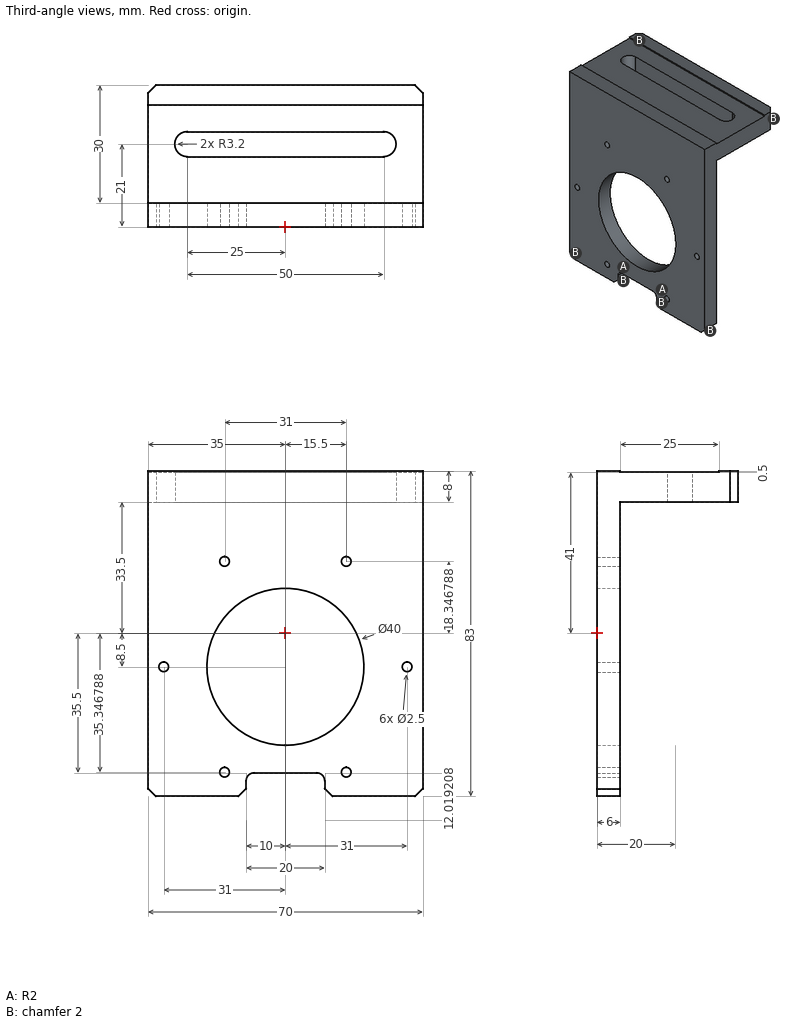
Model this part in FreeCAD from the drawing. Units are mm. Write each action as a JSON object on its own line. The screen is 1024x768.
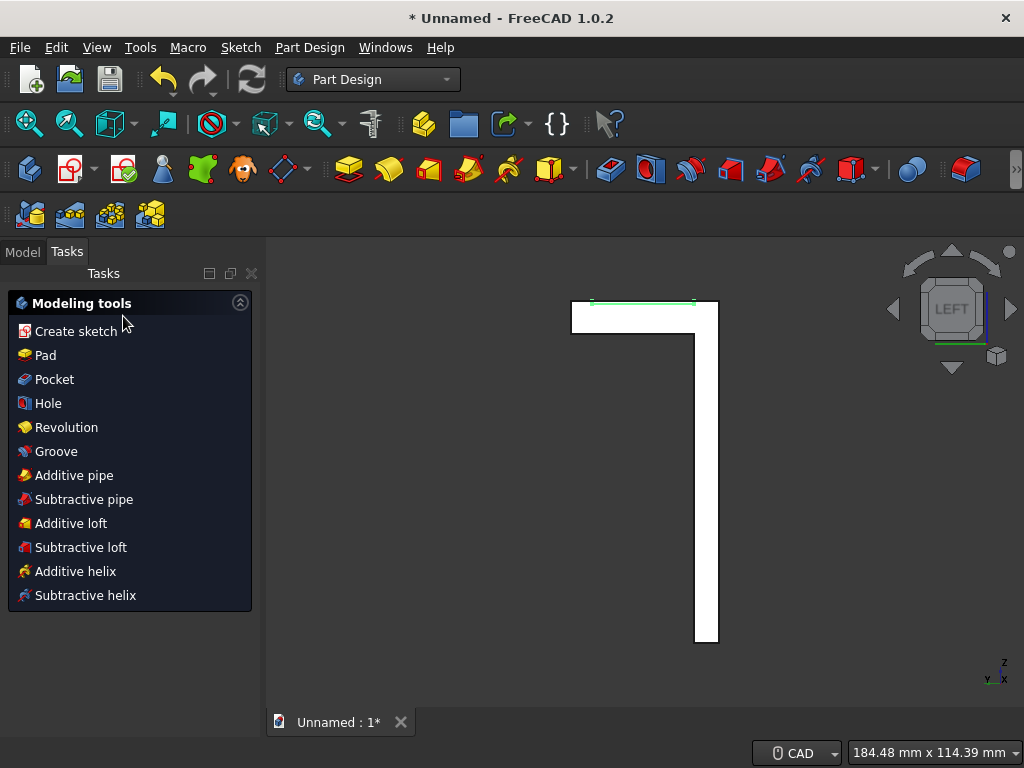
{"action": "left_click", "coordinate": [612, 170]}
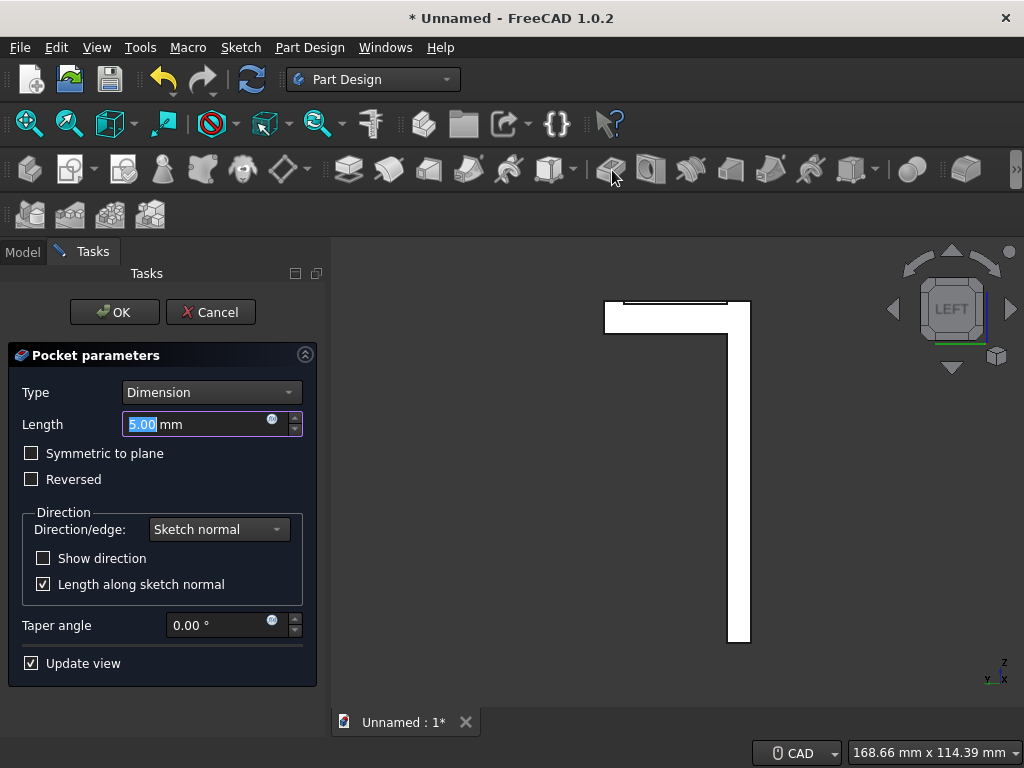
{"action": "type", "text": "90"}
{"action": "key", "text": "Tab"}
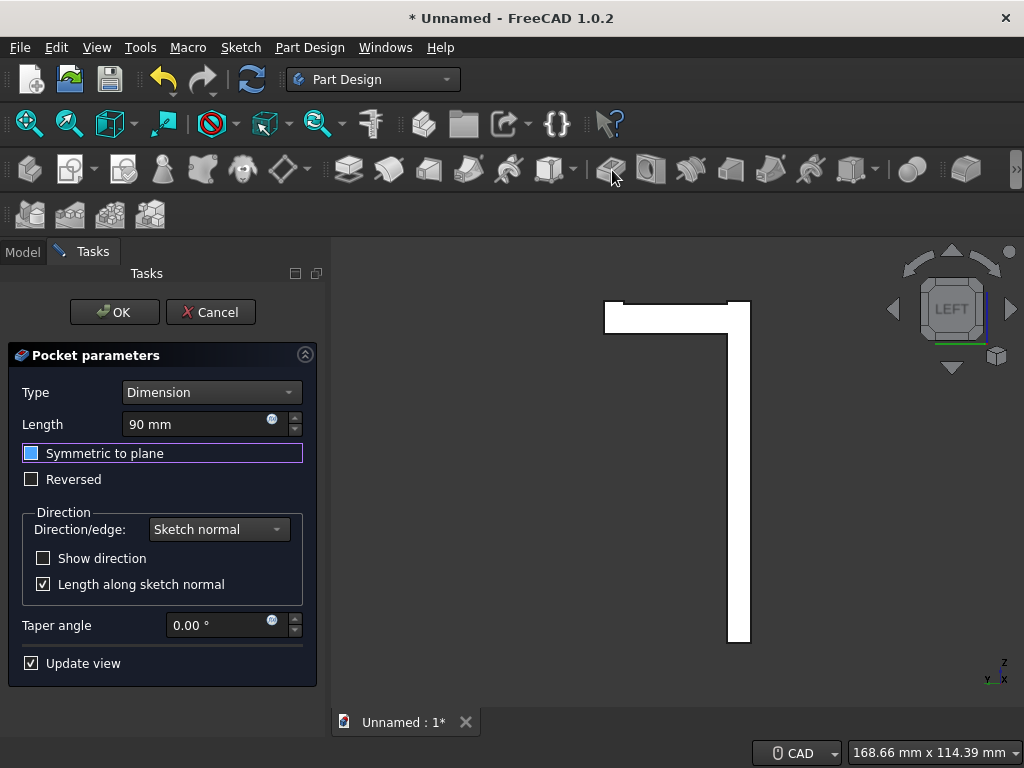
{"action": "left_click", "coordinate": [115, 312]}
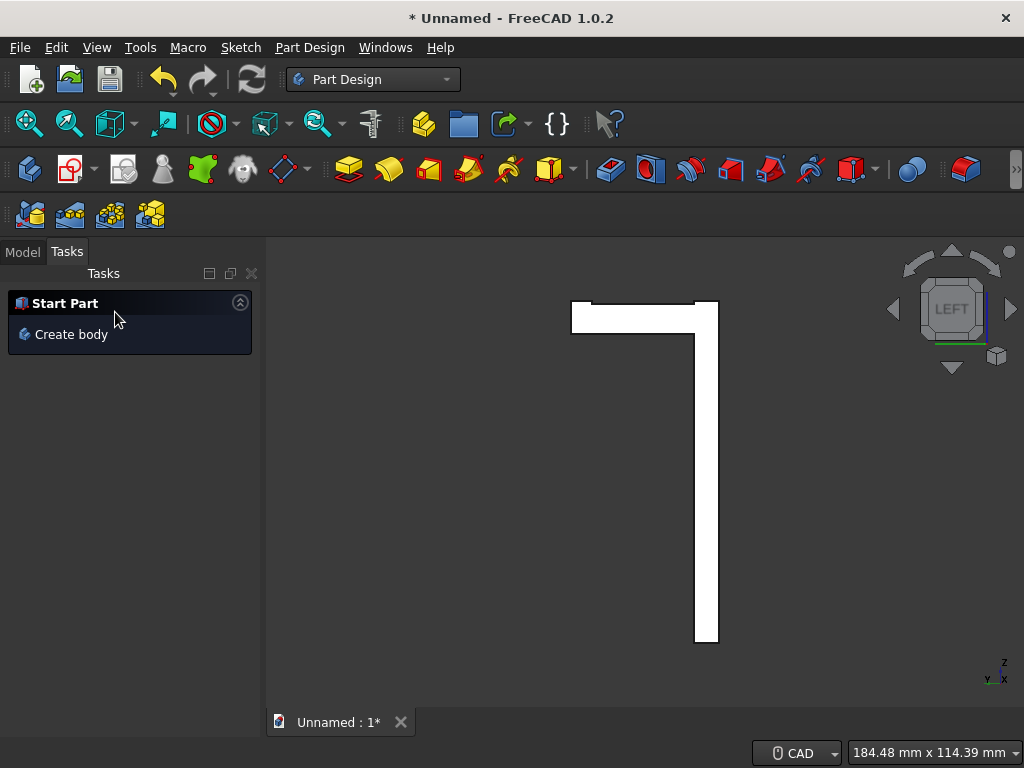
{"action": "key", "text": "0"}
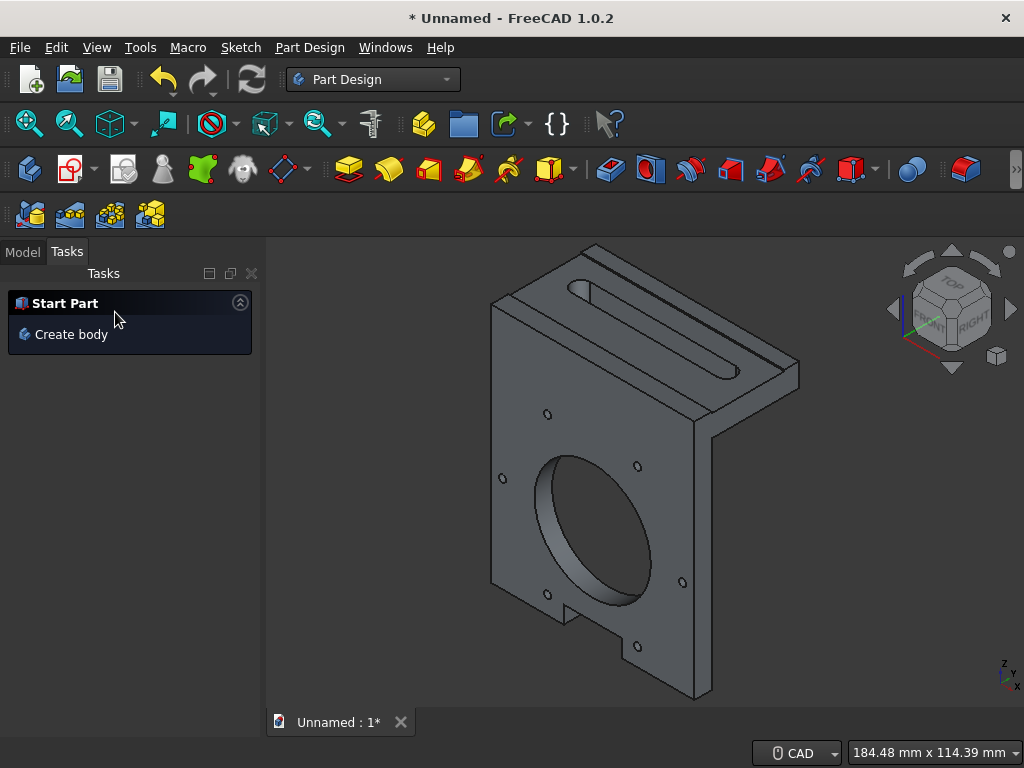
{"action": "key", "text": "2"}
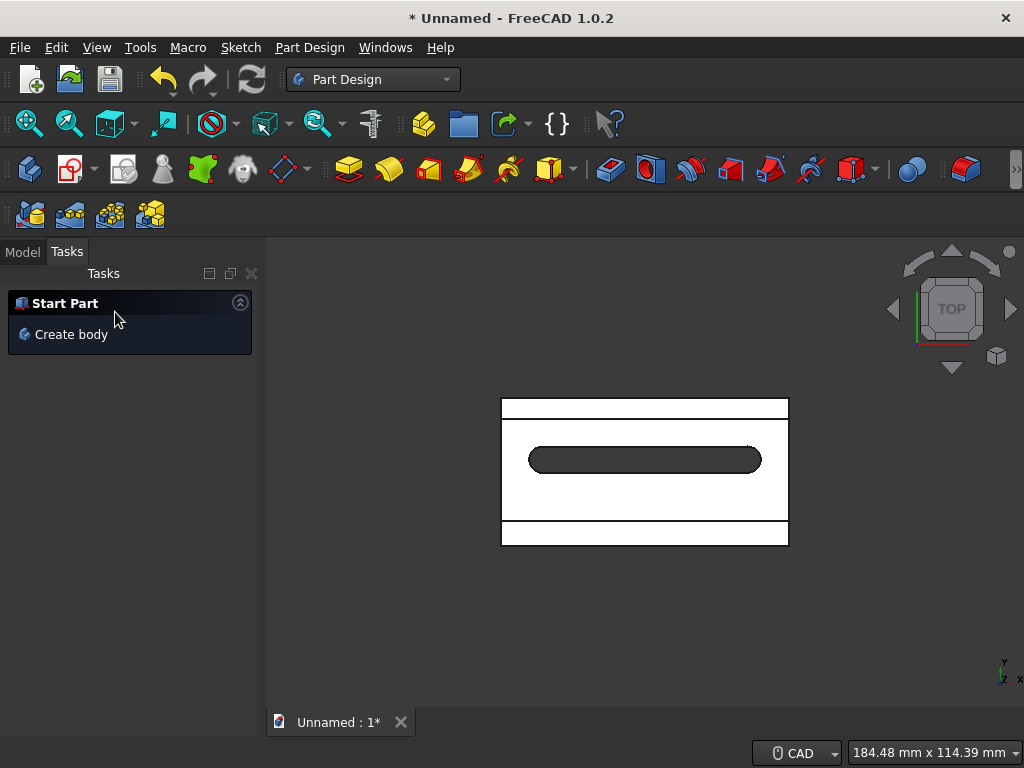
{"action": "left_click", "coordinate": [30, 124]}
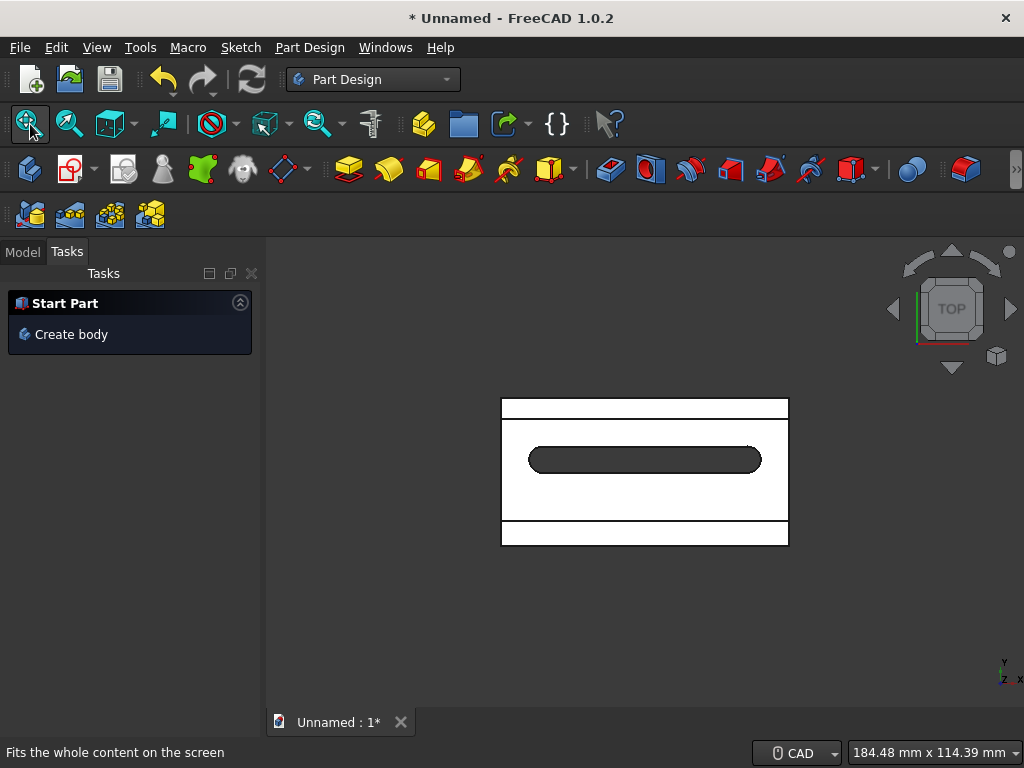
{"action": "key", "text": "1"}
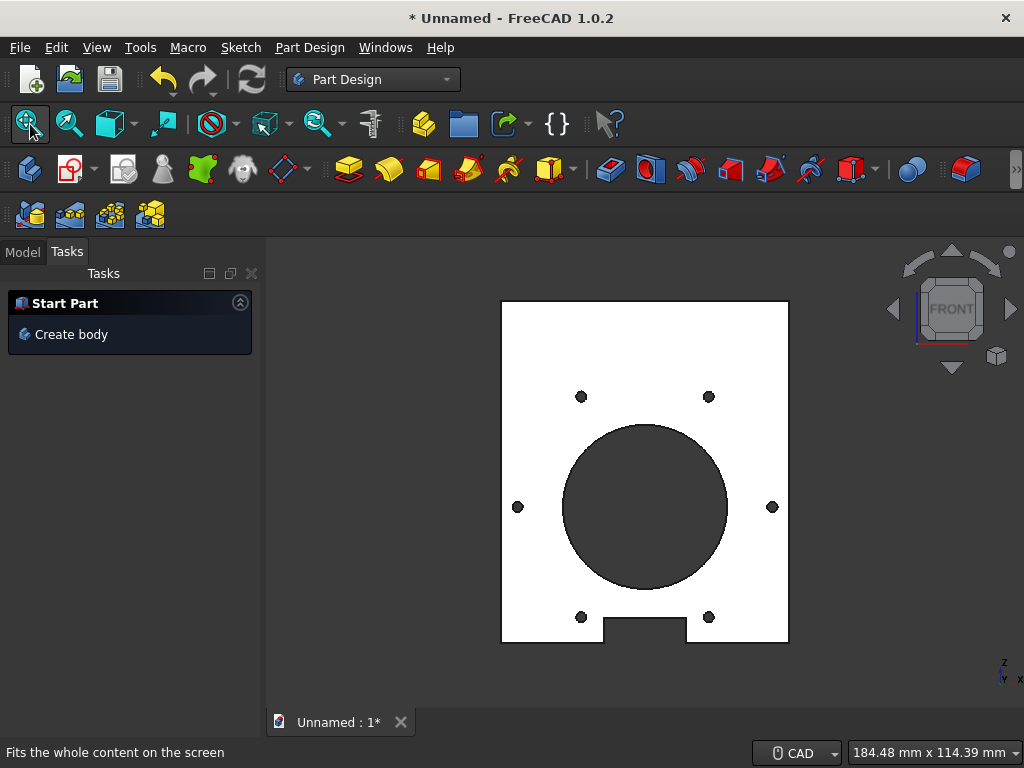
{"action": "key", "text": "3"}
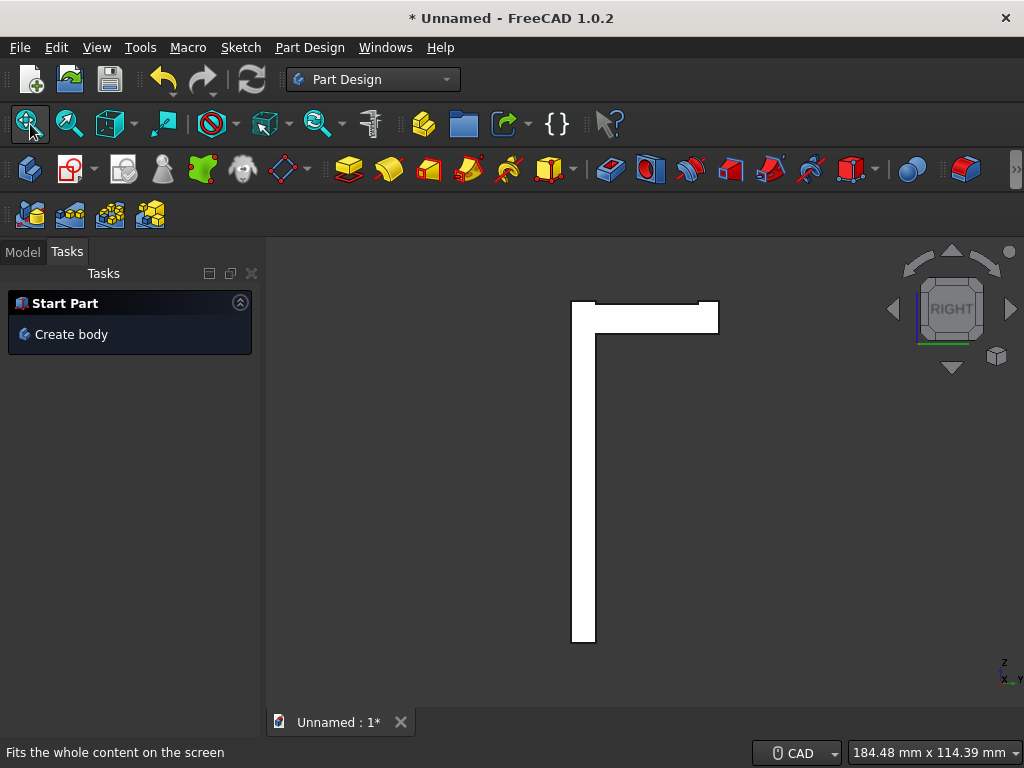
{"action": "key", "text": "5"}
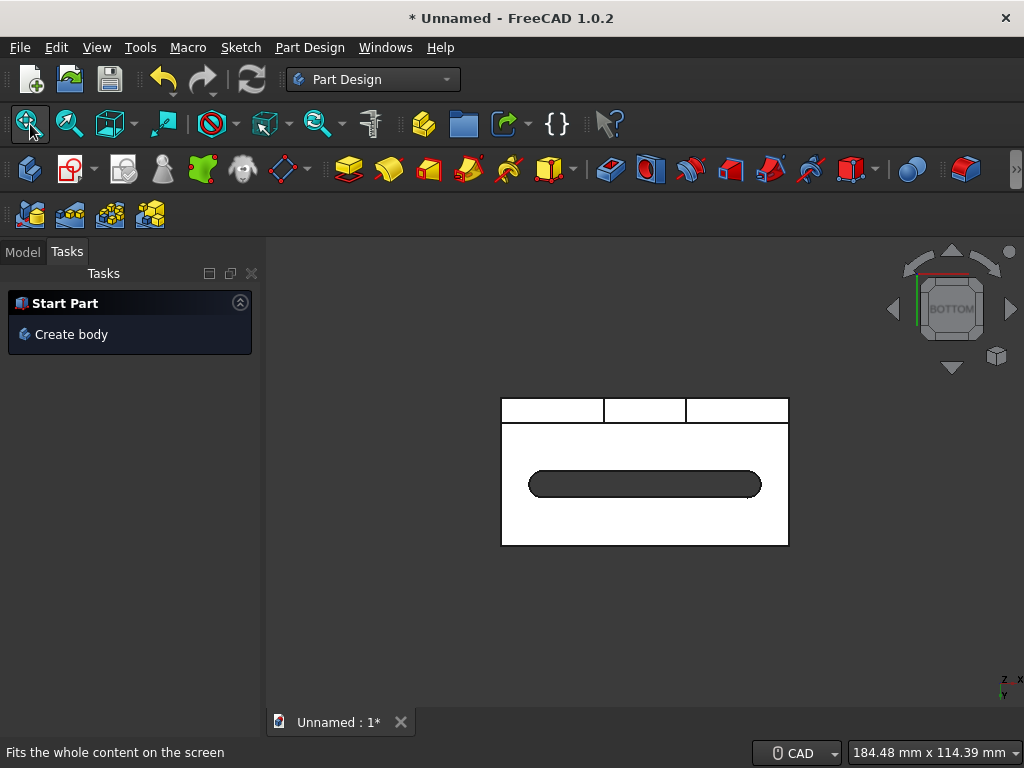
{"action": "left_click", "coordinate": [30, 124]}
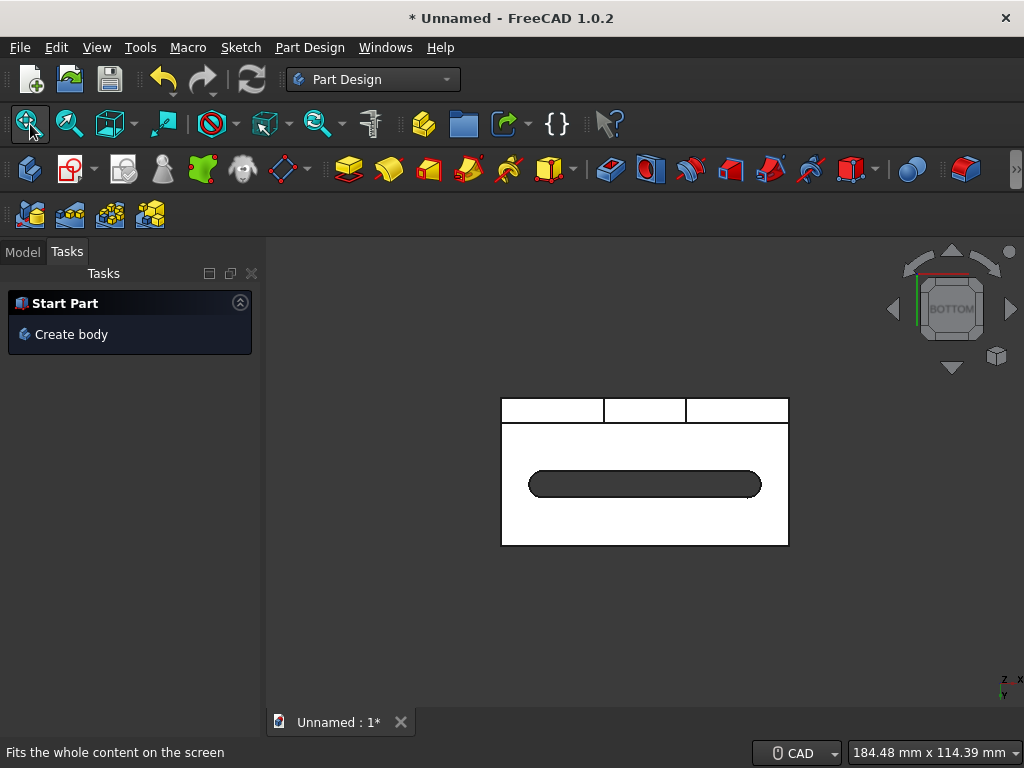
{"action": "key", "text": "4"}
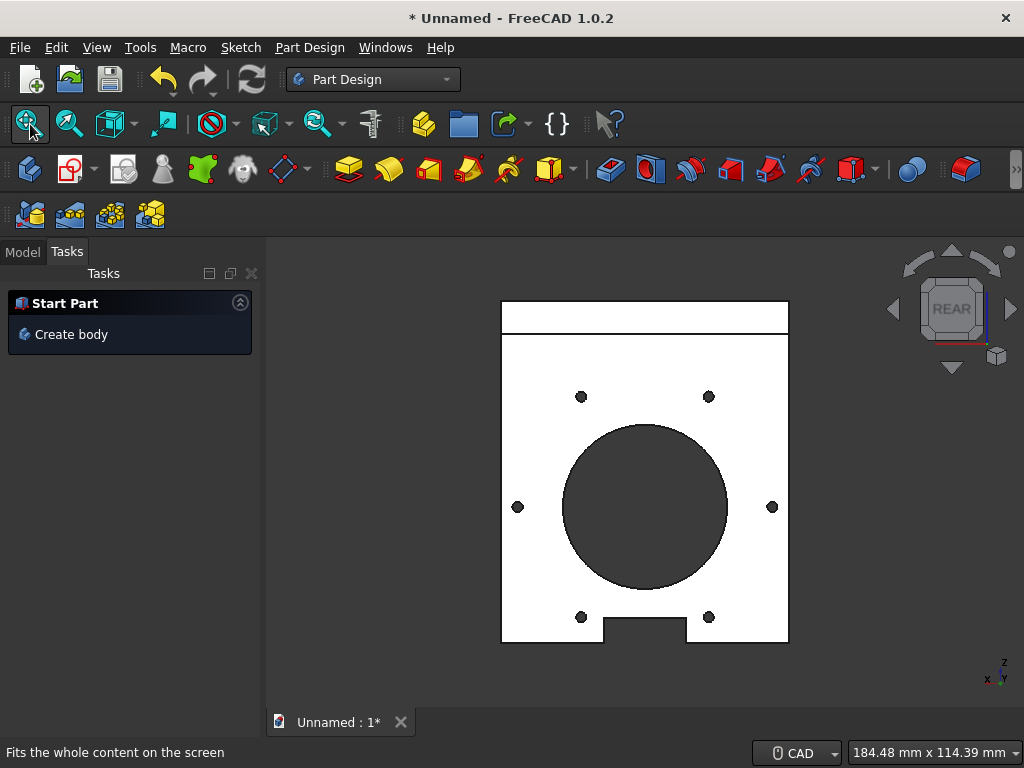
{"action": "key", "text": "6"}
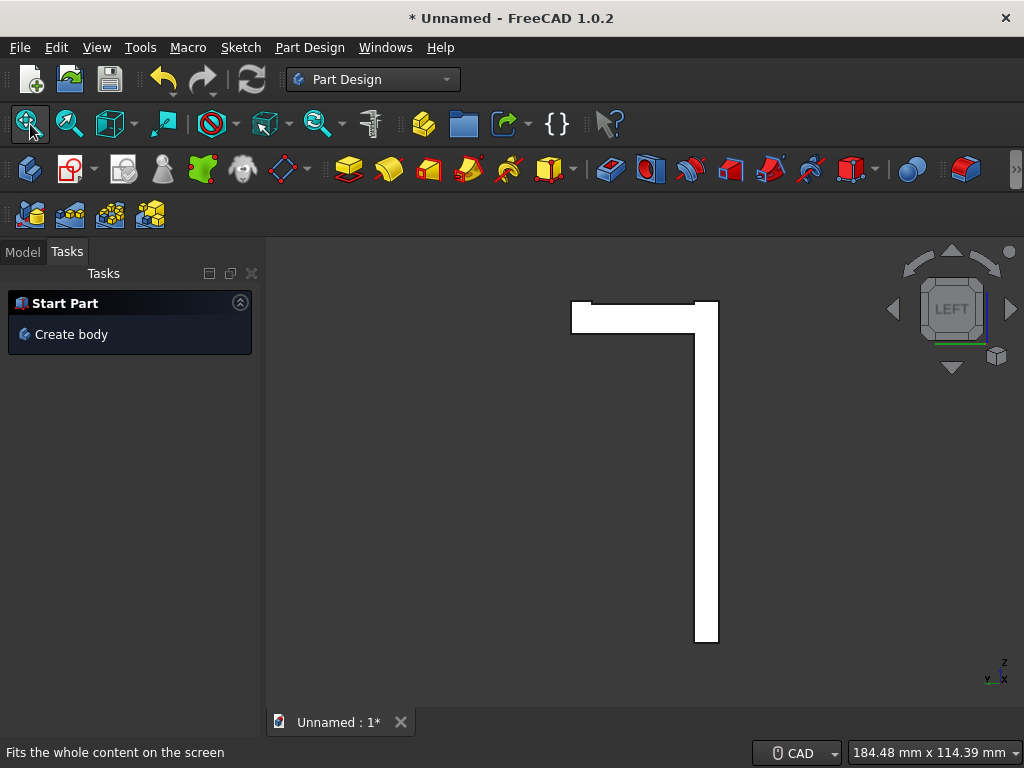
{"action": "key", "text": "v 3"}